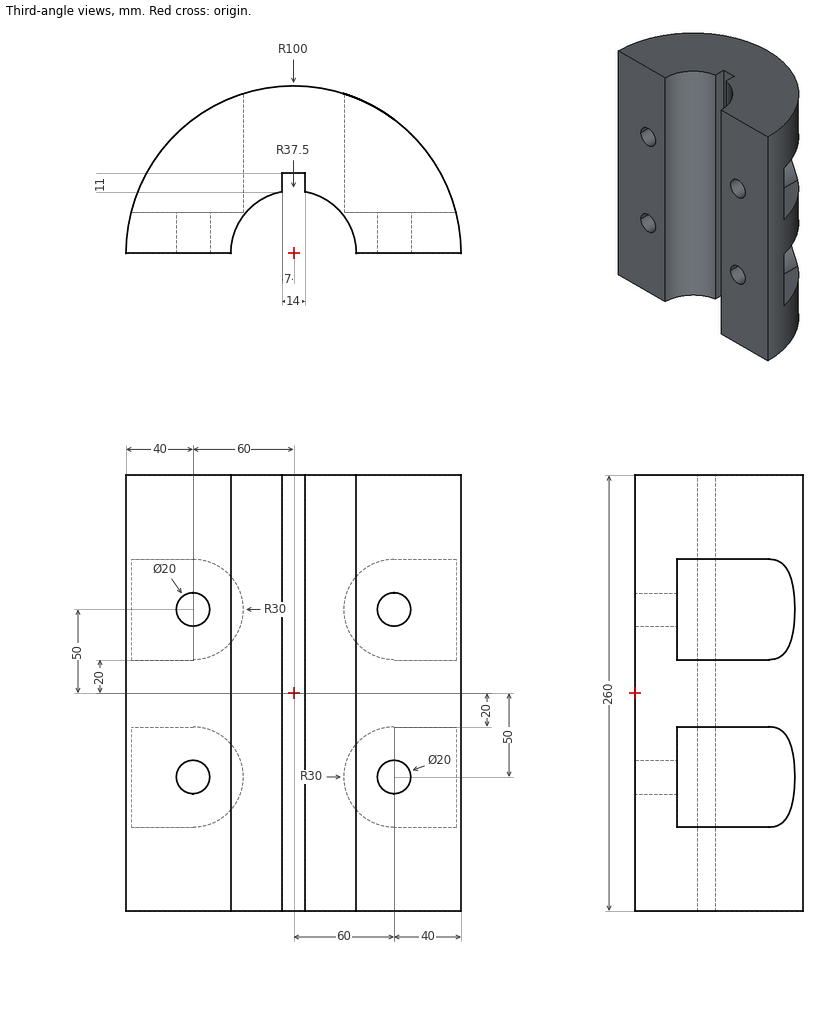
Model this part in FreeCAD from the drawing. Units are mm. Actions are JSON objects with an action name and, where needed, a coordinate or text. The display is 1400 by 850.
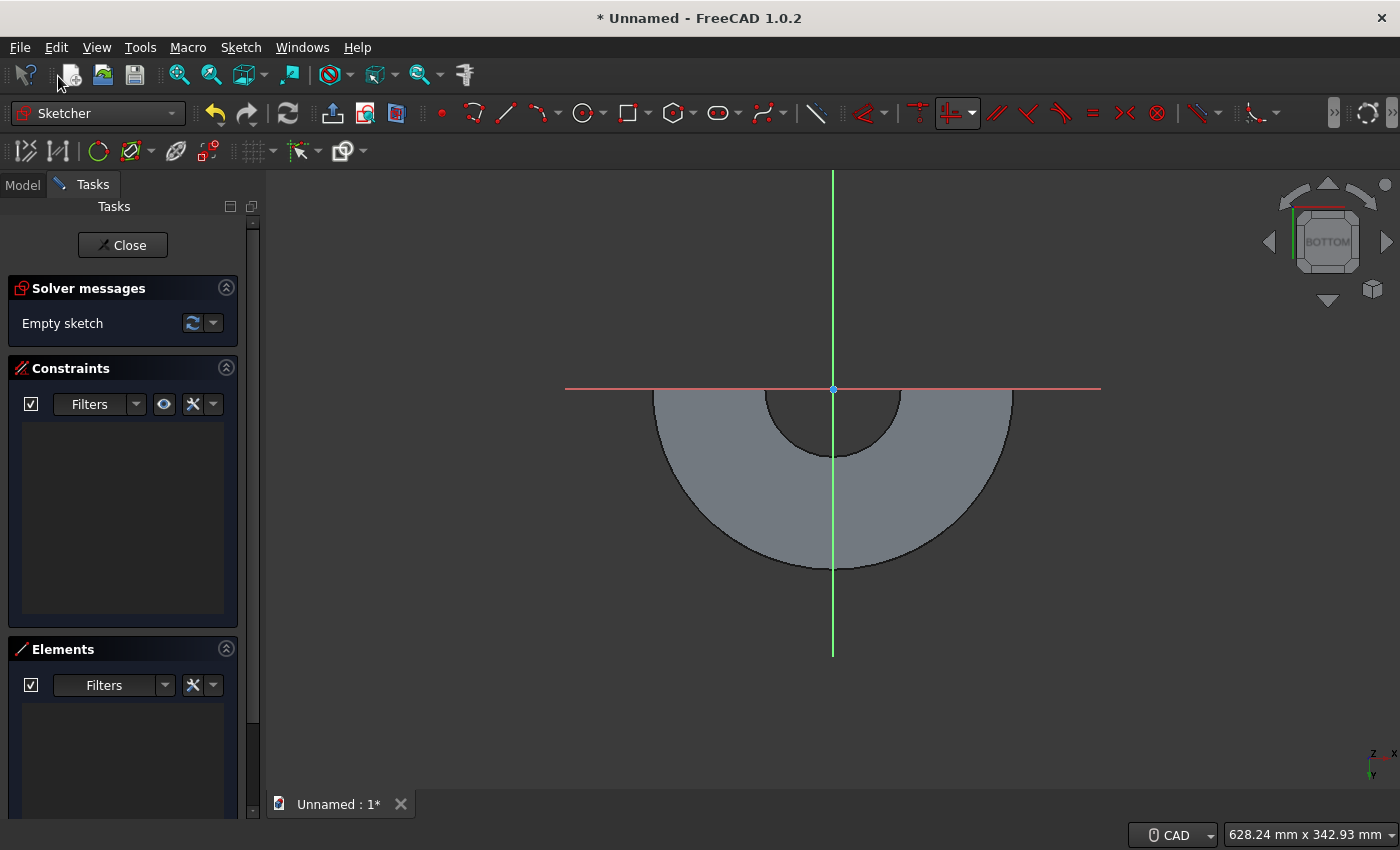
{"action": "scroll", "coordinate": [837, 465], "scroll_direction": "up", "scroll_amount": 15}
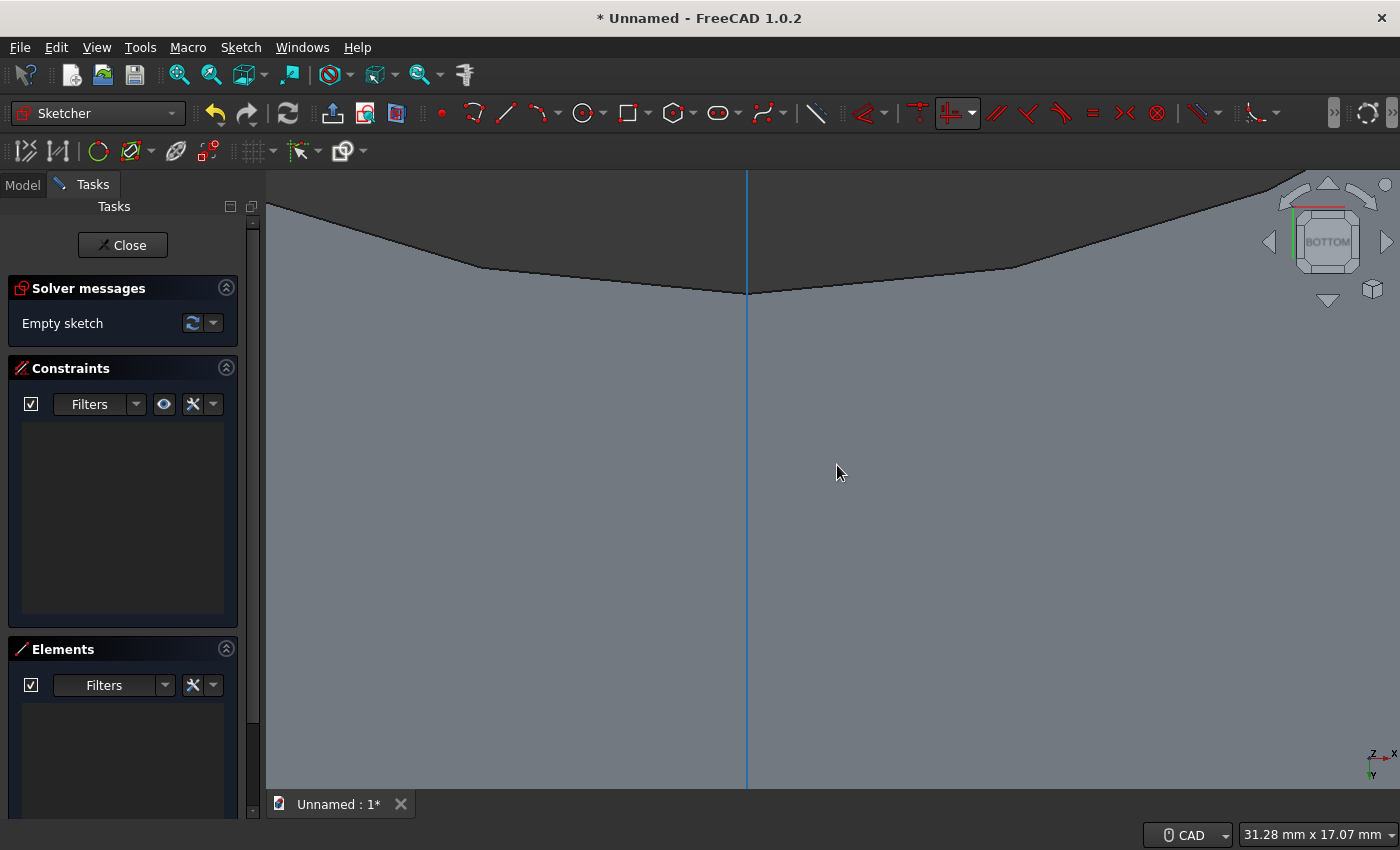
{"action": "left_click", "coordinate": [474, 114]}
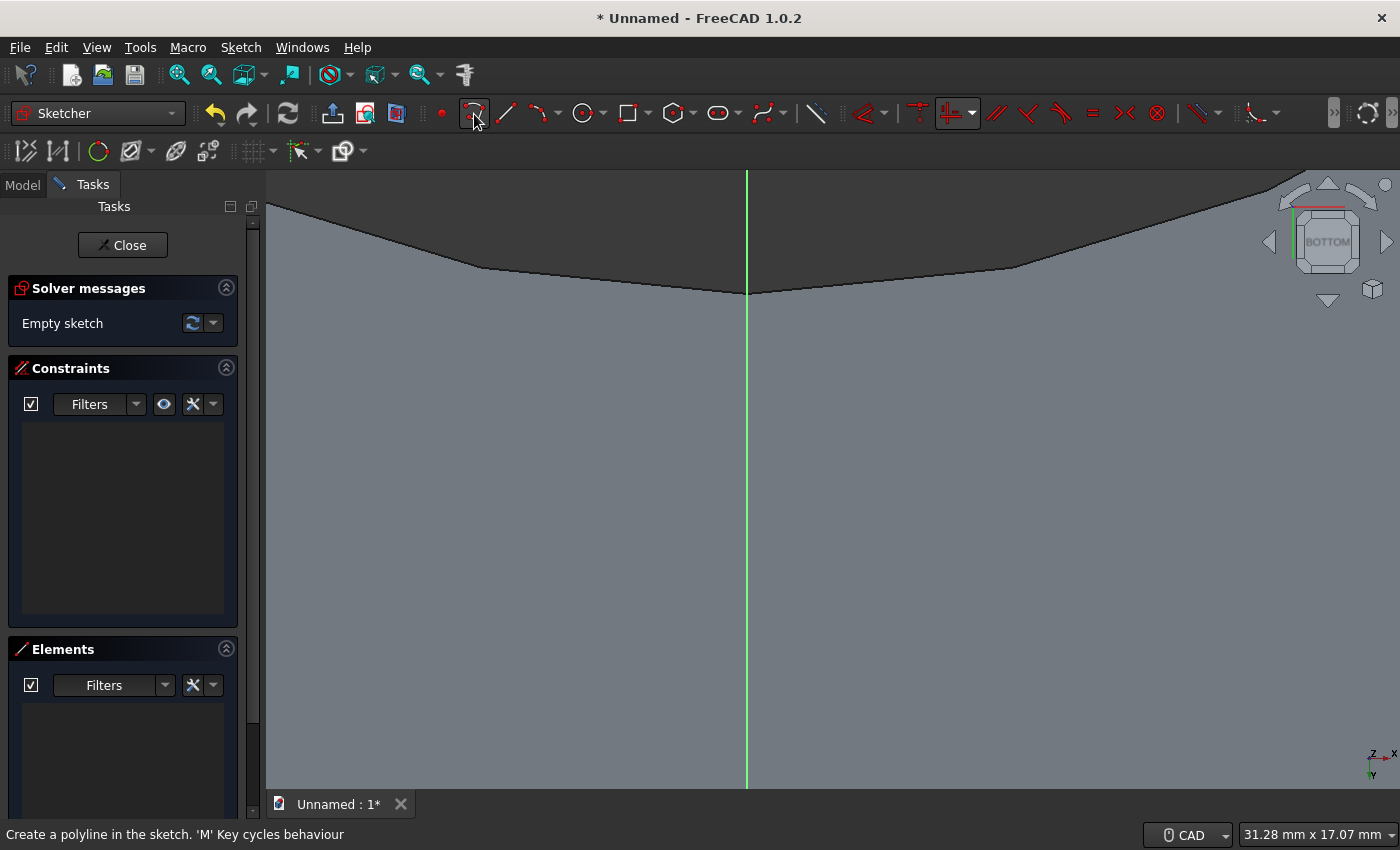
{"action": "left_click", "coordinate": [493, 270]}
{"action": "left_click", "coordinate": [493, 669]}
{"action": "left_click", "coordinate": [1001, 669]}
{"action": "left_click", "coordinate": [1001, 270]}
{"action": "right_click", "coordinate": [1001, 270]}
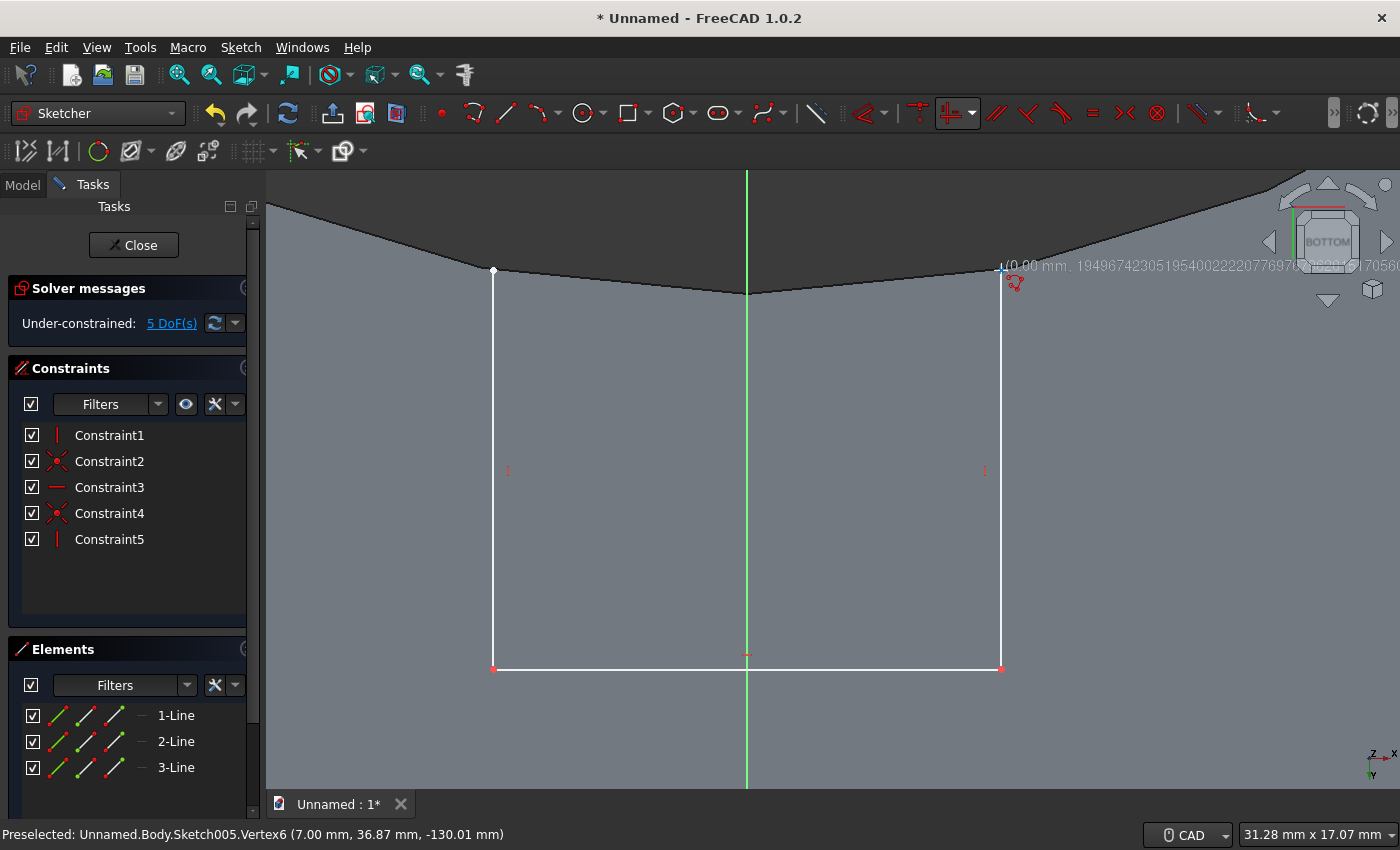
{"action": "left_click", "coordinate": [538, 114]}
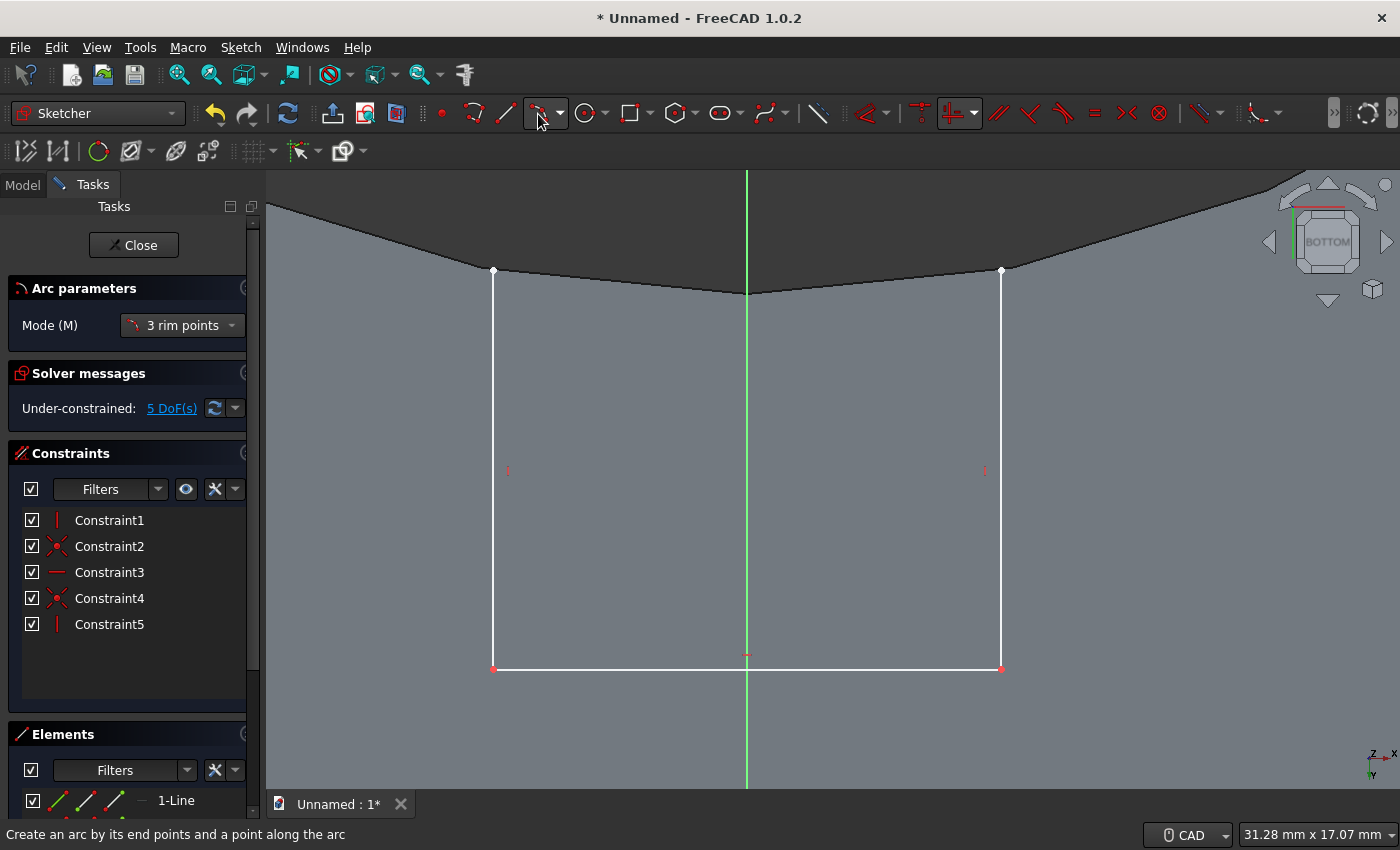
{"action": "left_click", "coordinate": [1001, 271]}
{"action": "left_click", "coordinate": [493, 271]}
{"action": "left_click", "coordinate": [696, 293]}
{"action": "key", "text": "Escape"}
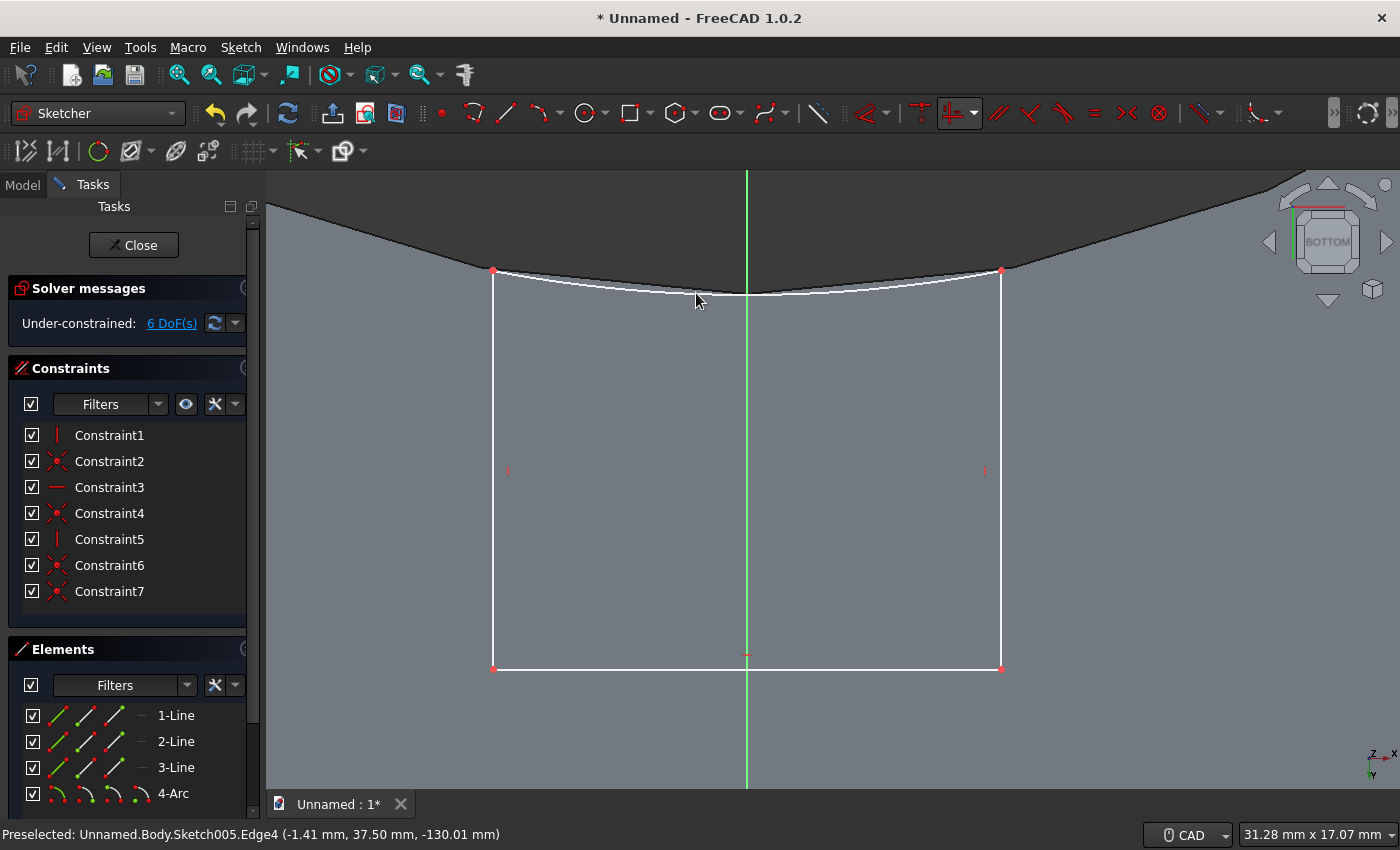
{"action": "scroll", "coordinate": [770, 701], "scroll_direction": "down", "scroll_amount": 7}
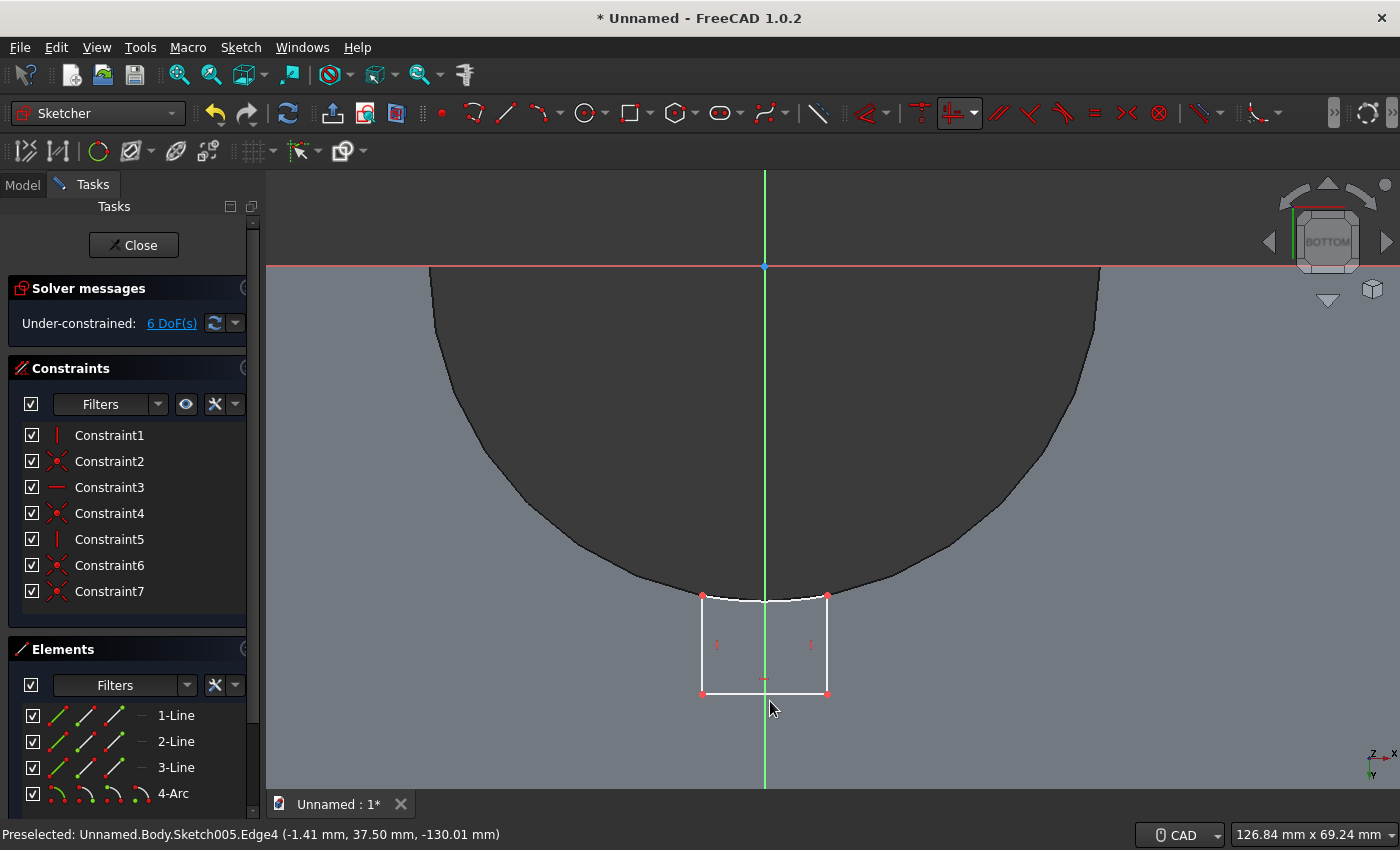
{"action": "left_click_drag", "start_coordinate": [755, 256], "coordinate": [775, 277]}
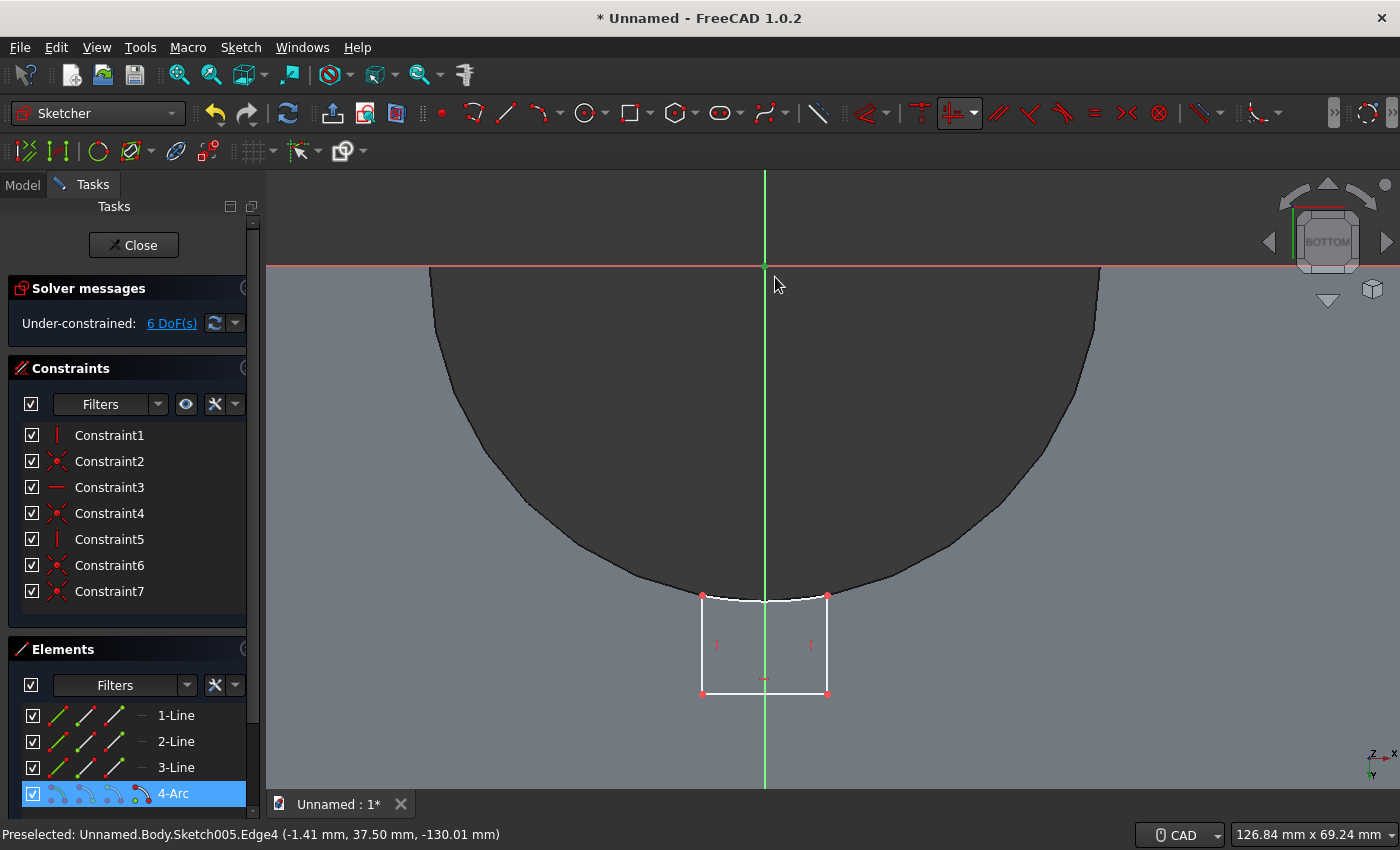
{"action": "left_click", "coordinate": [920, 114]}